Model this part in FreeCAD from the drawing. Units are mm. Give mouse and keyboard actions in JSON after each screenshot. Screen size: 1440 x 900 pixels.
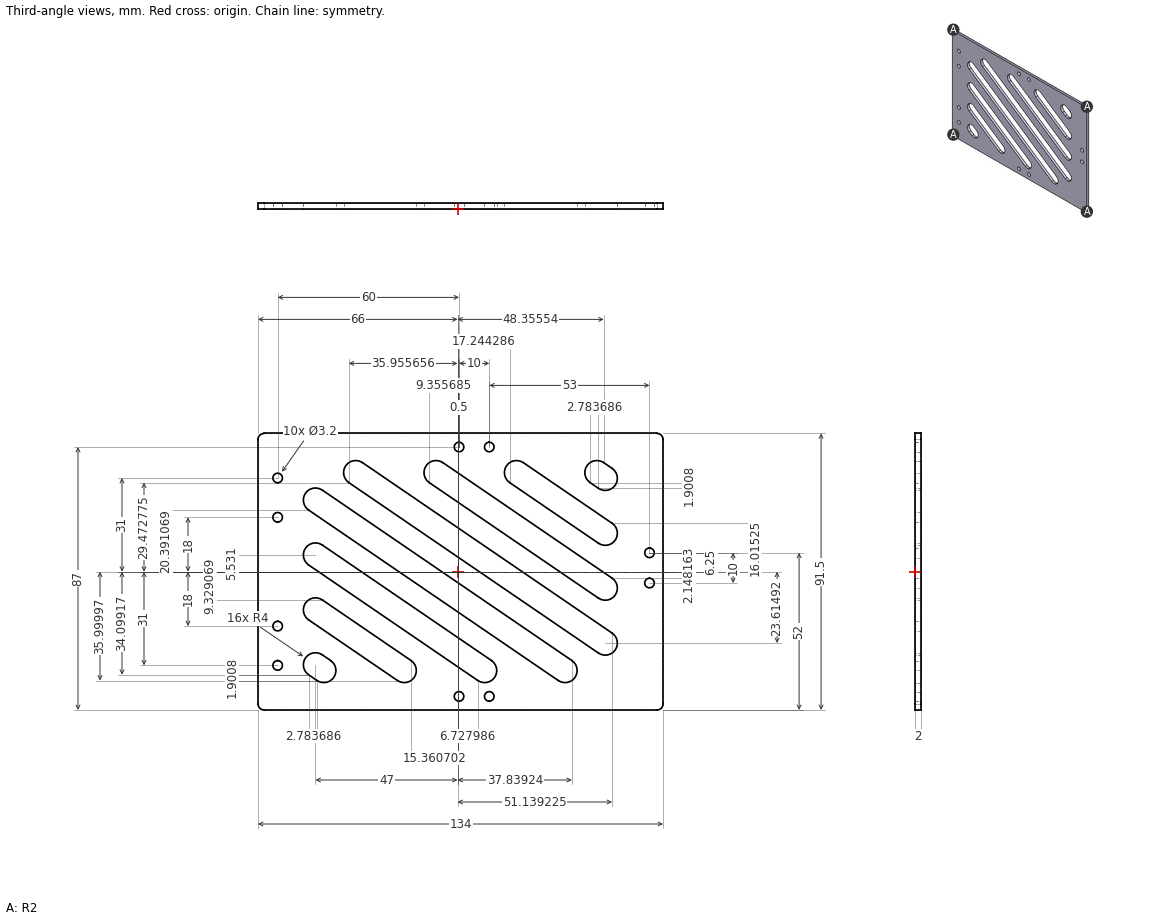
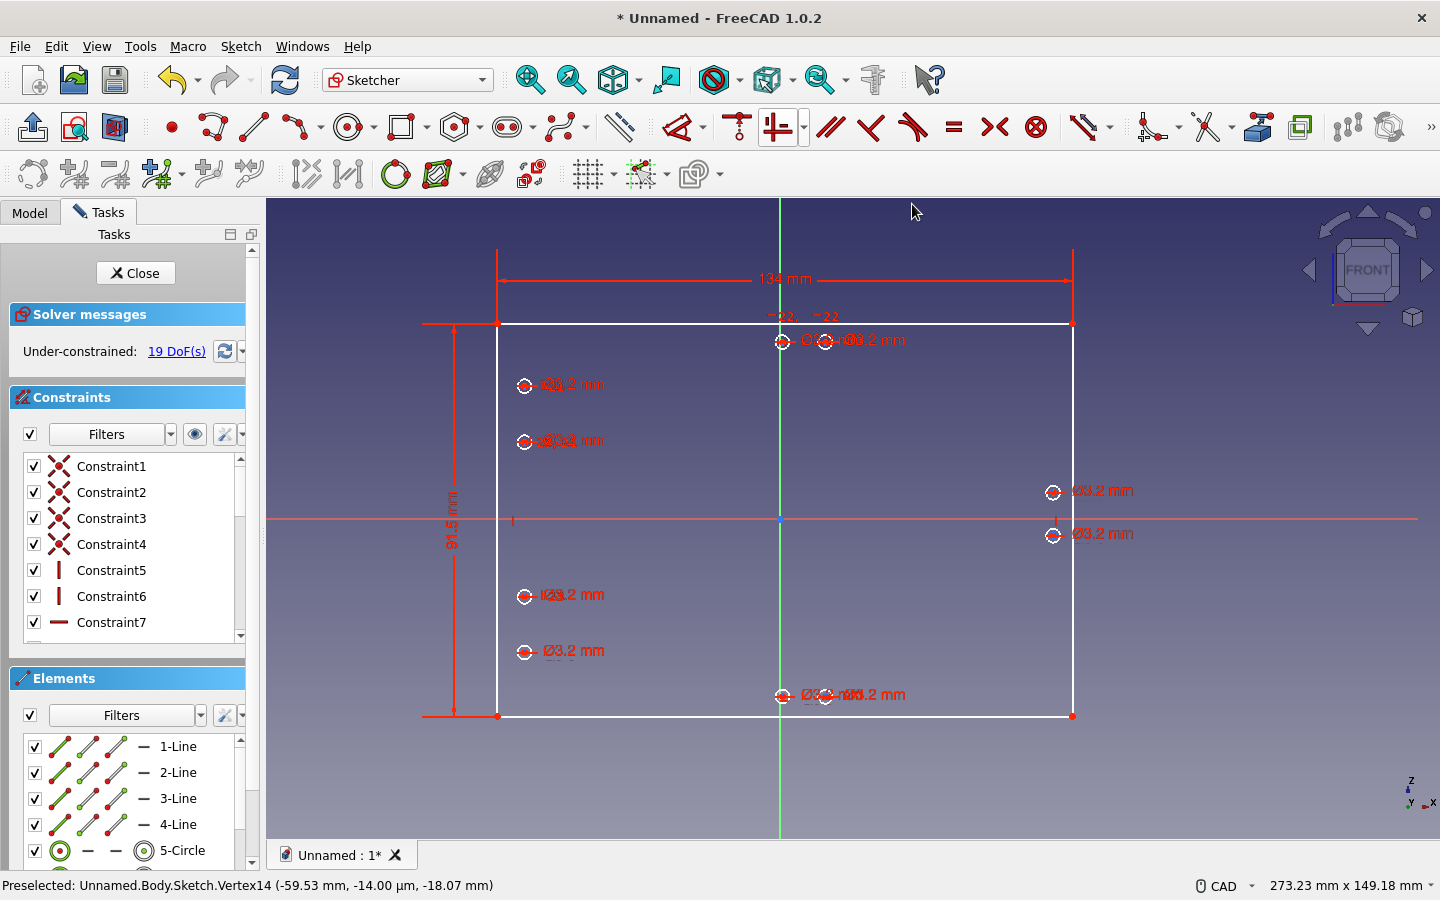
{"action": "left_click", "coordinate": [525, 597]}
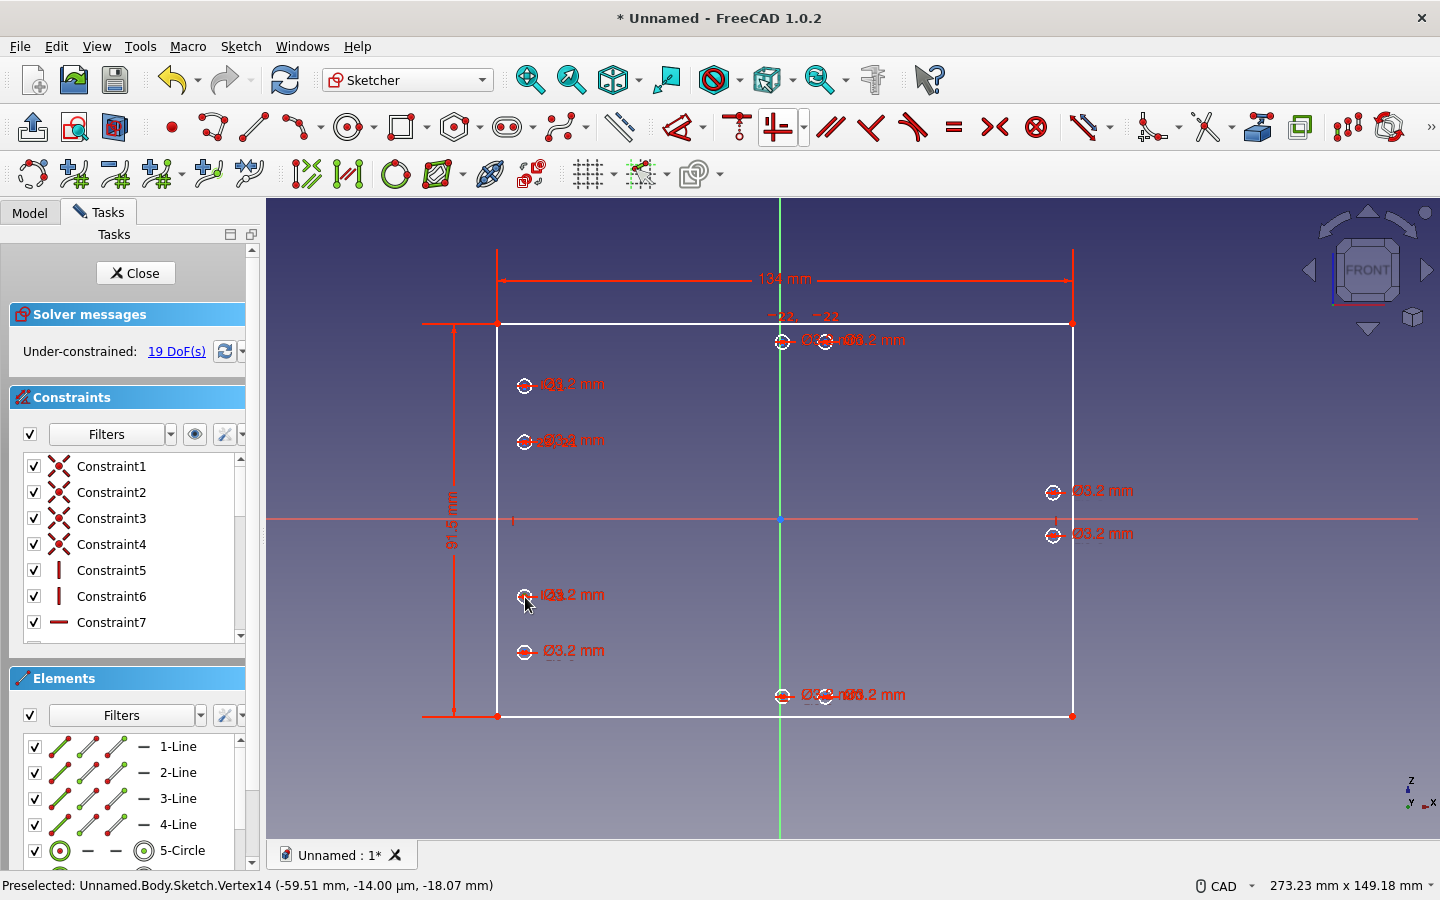
{"action": "left_click", "coordinate": [524, 653]}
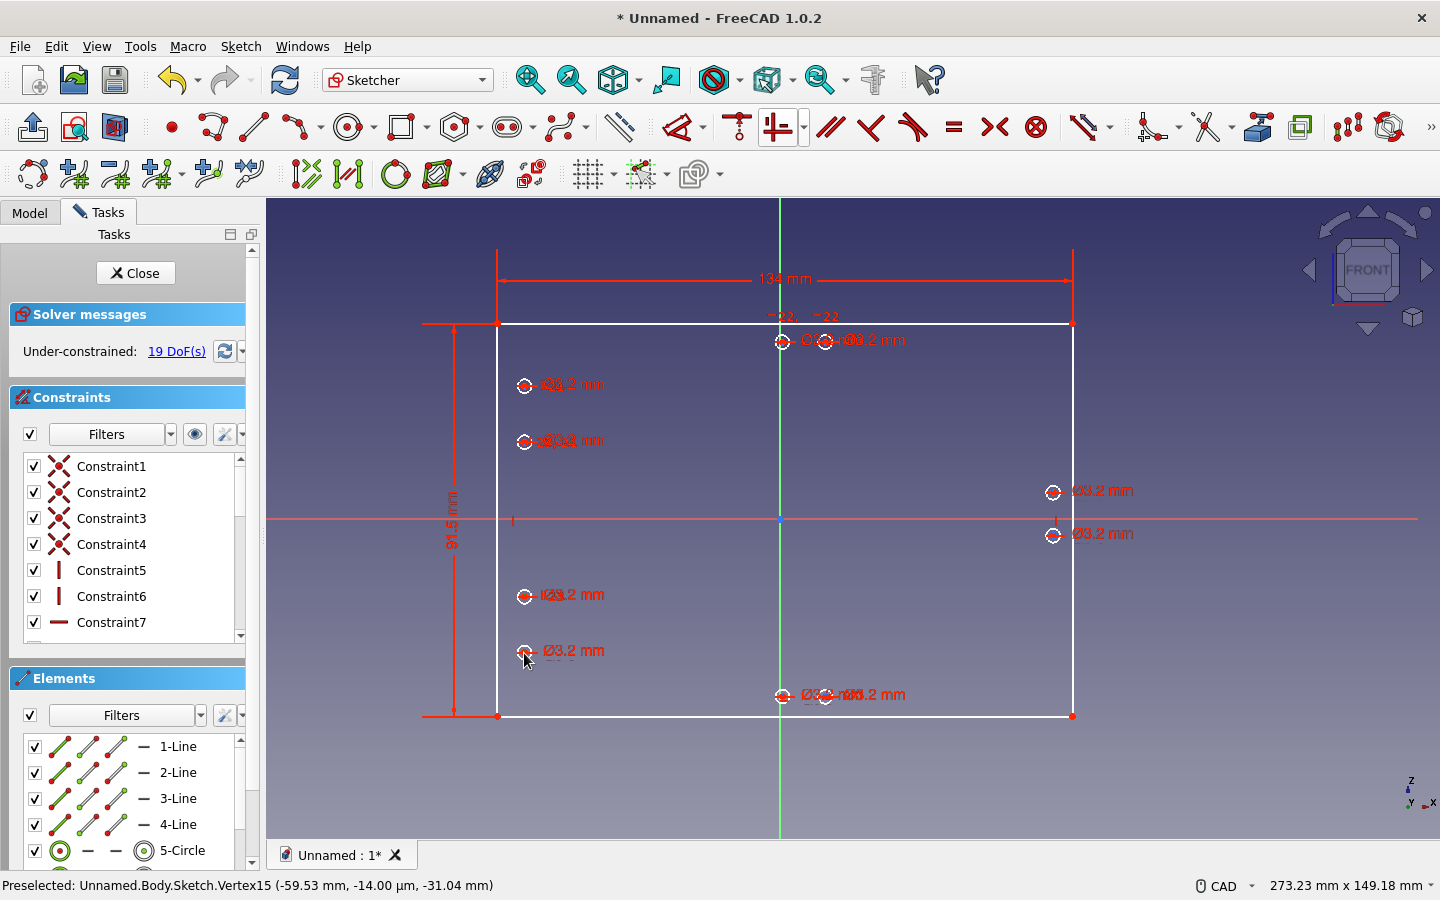
{"action": "left_click", "coordinate": [804, 128]}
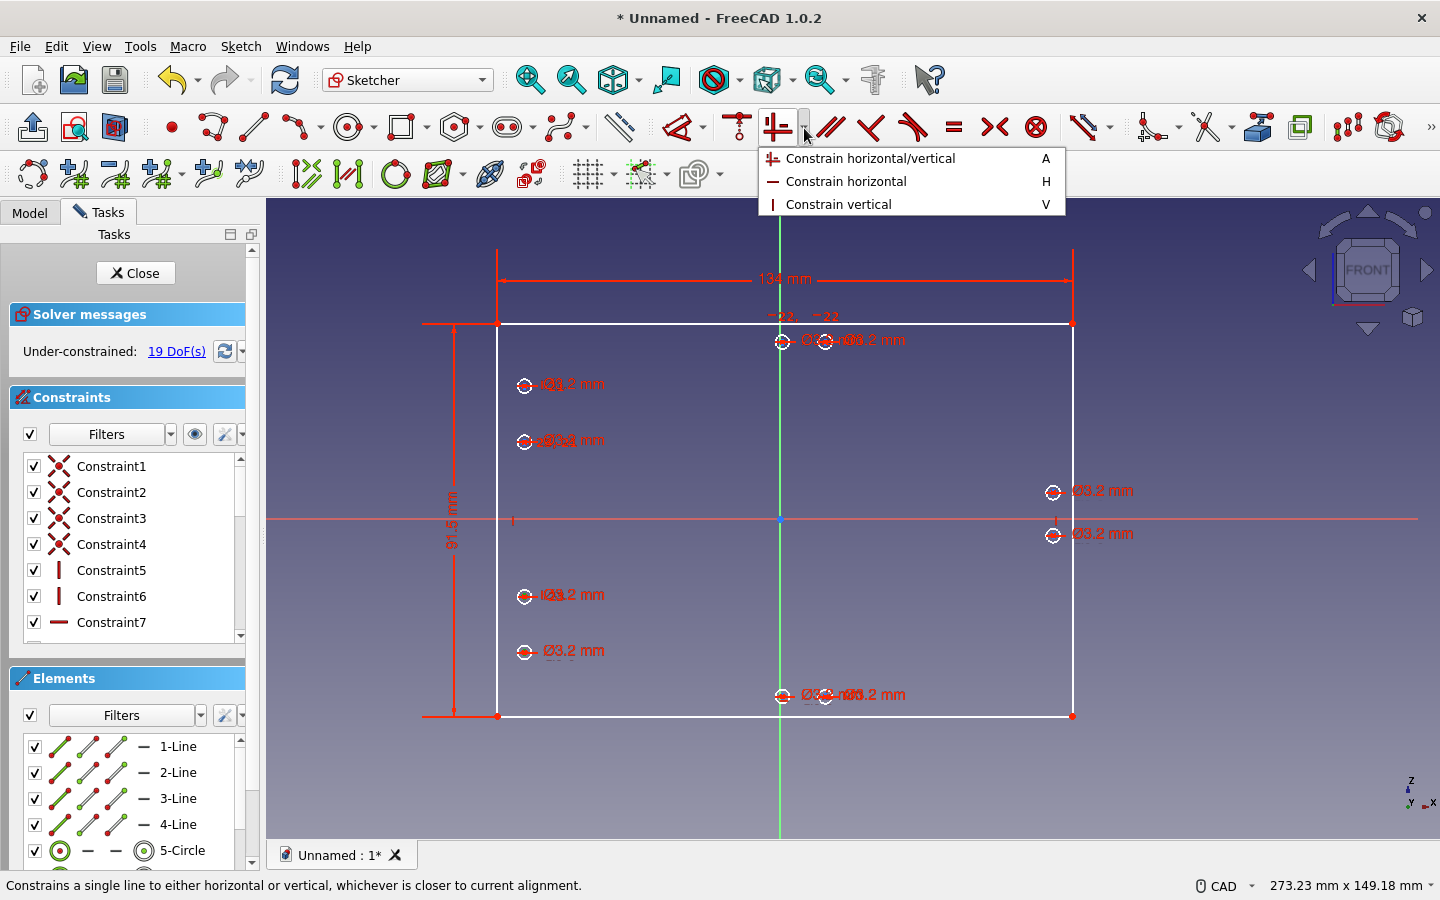
{"action": "left_click", "coordinate": [912, 204]}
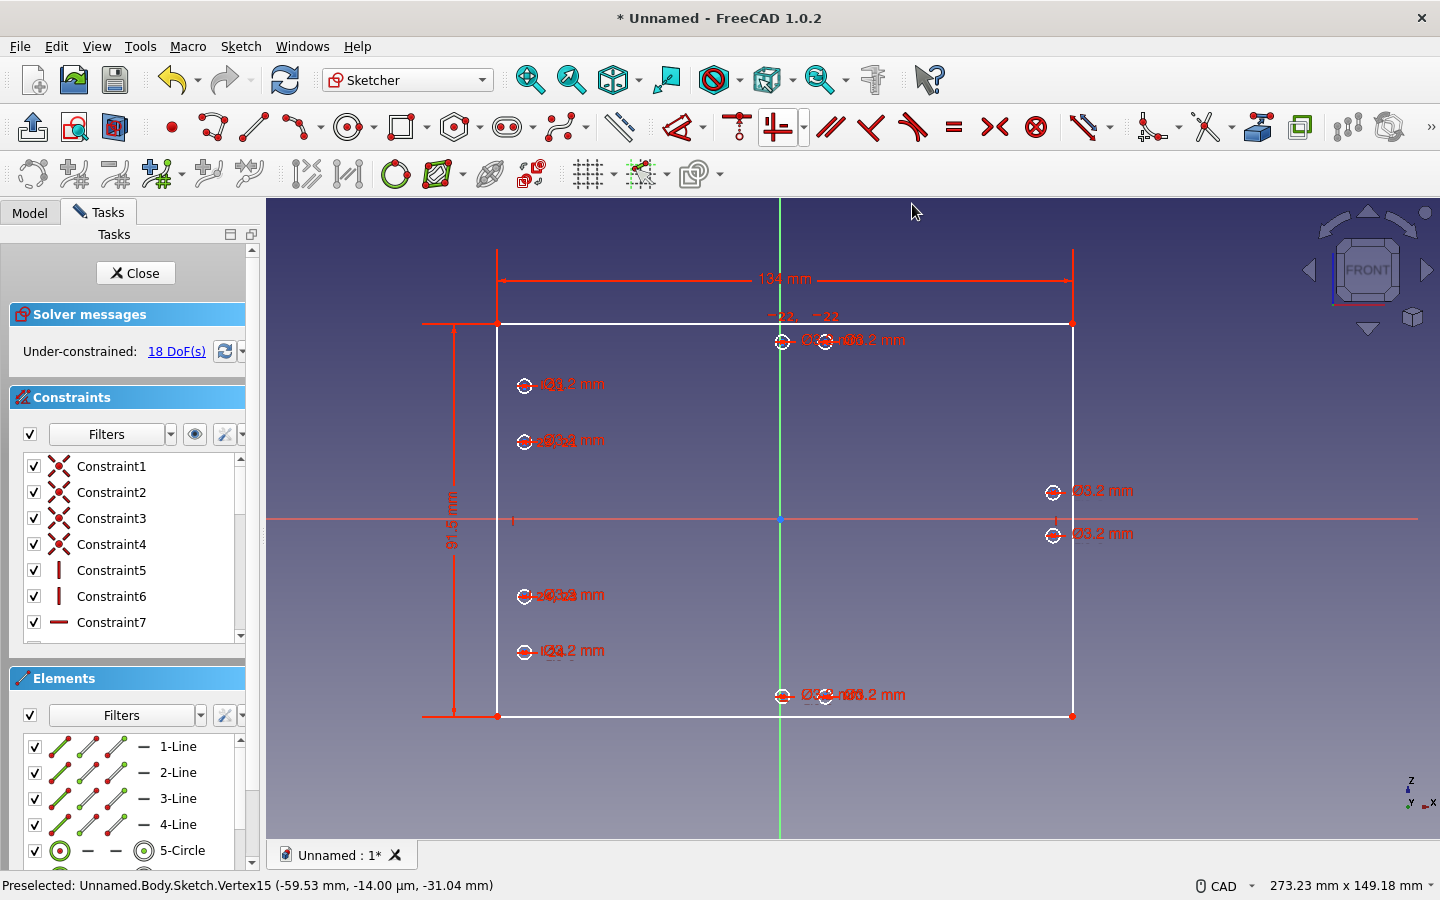
{"action": "left_click", "coordinate": [1053, 493]}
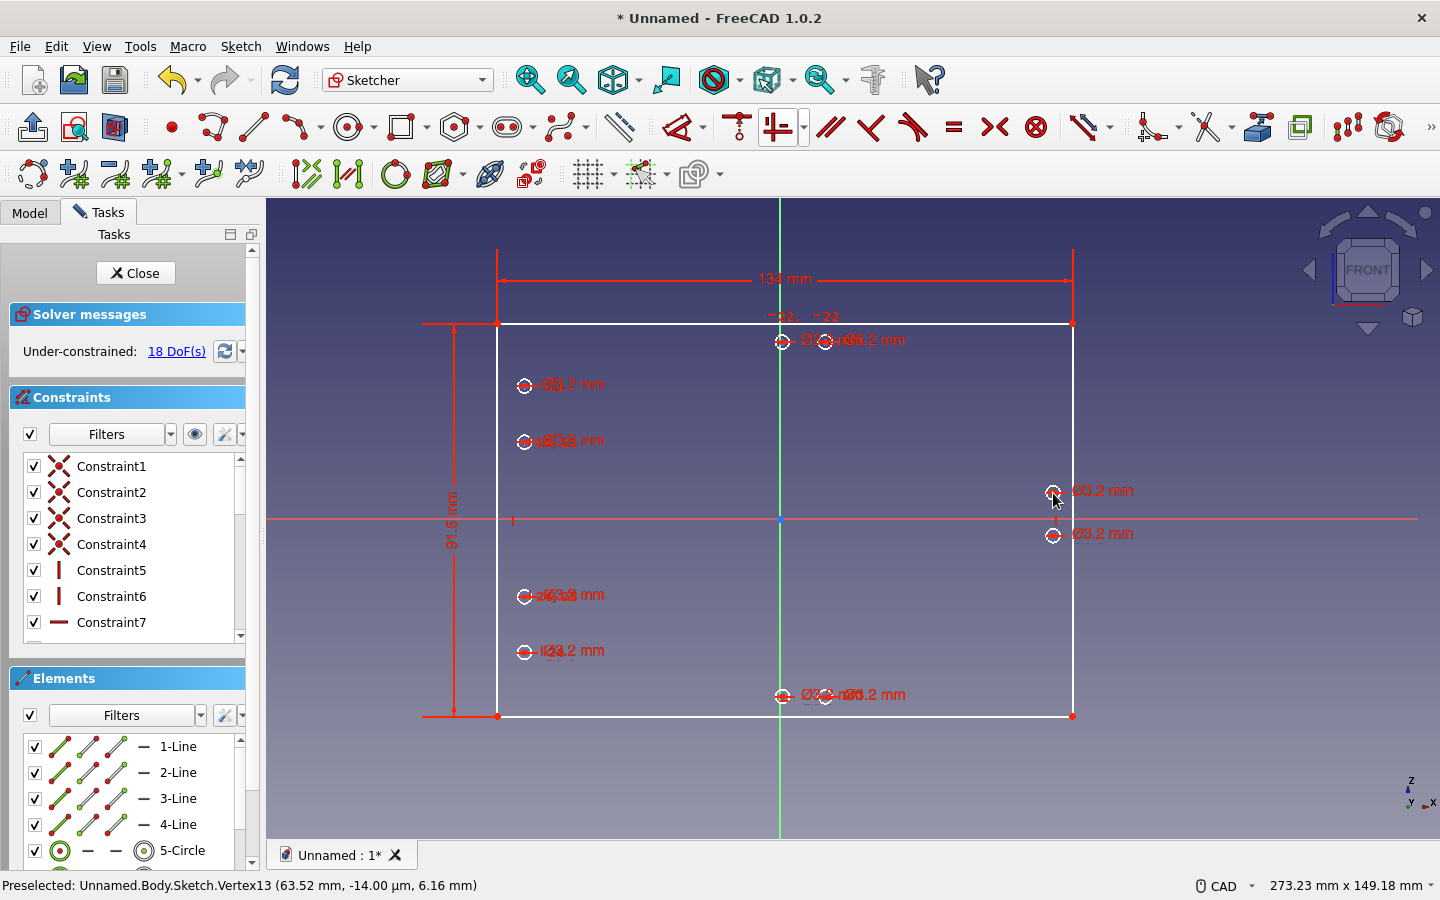
{"action": "left_click", "coordinate": [1053, 536]}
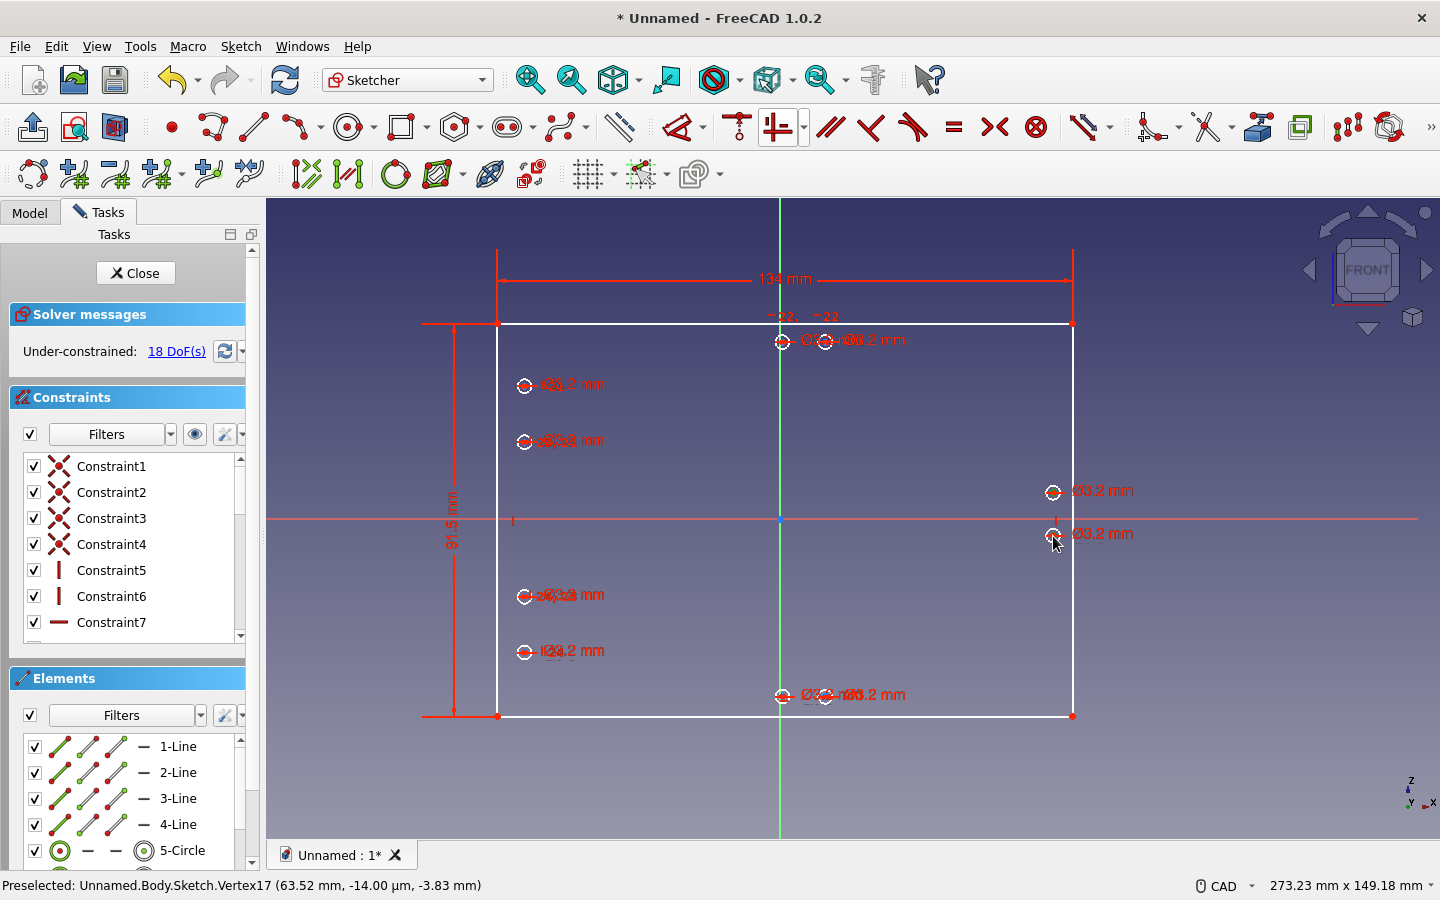
{"action": "left_click", "coordinate": [804, 128]}